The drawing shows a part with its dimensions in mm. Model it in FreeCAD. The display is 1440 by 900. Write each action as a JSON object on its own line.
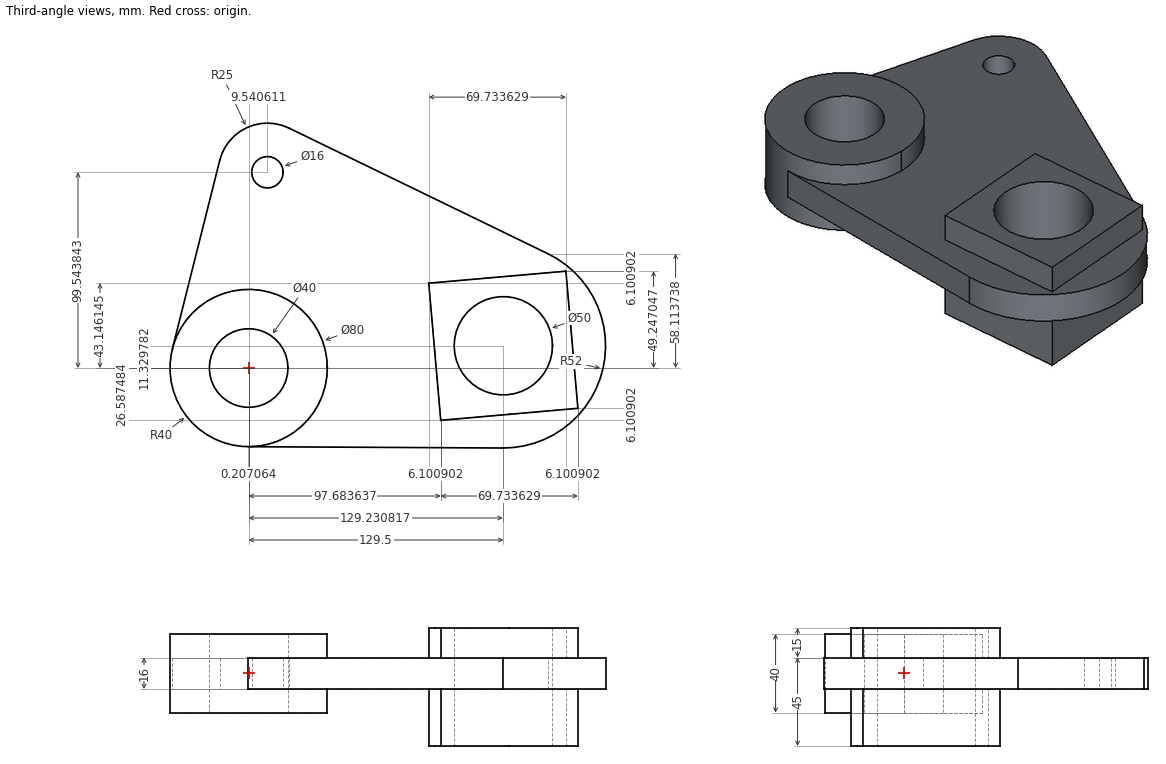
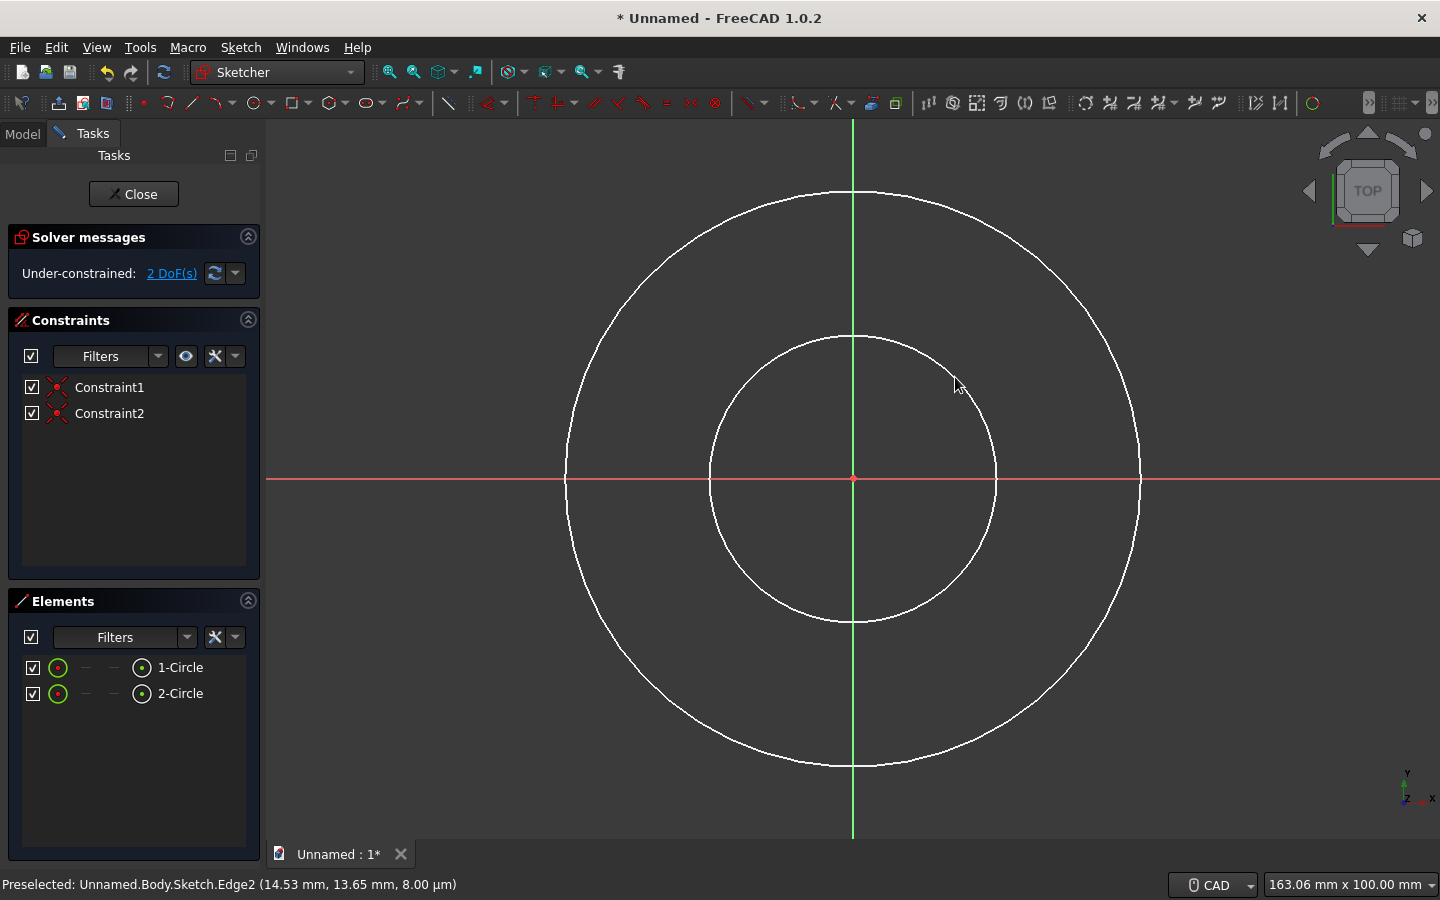
{"action": "key", "text": "d"}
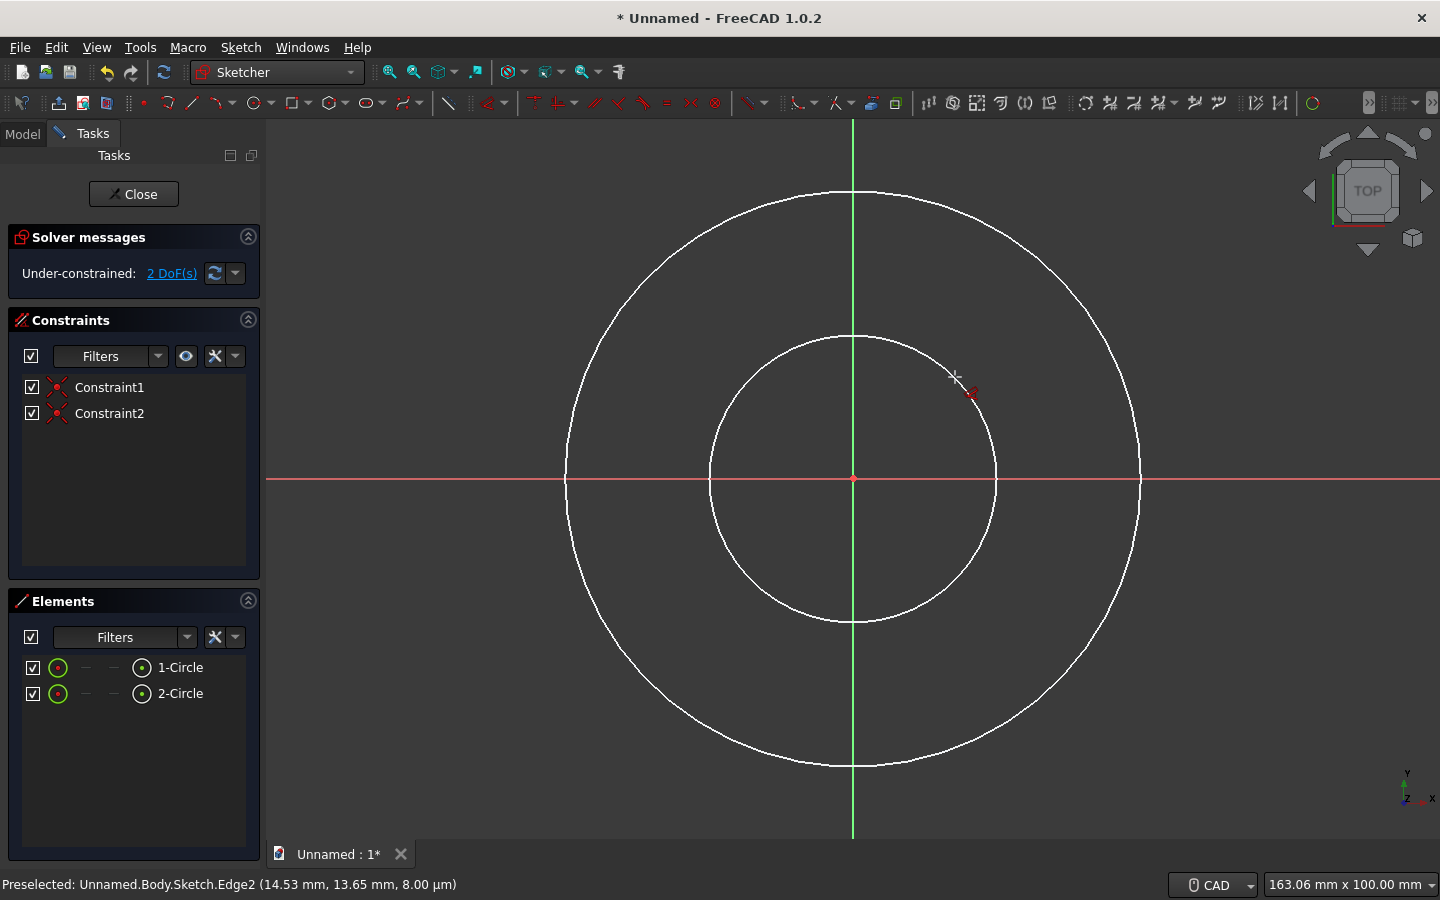
{"action": "left_click", "coordinate": [1056, 275]}
{"action": "left_click", "coordinate": [1079, 252]}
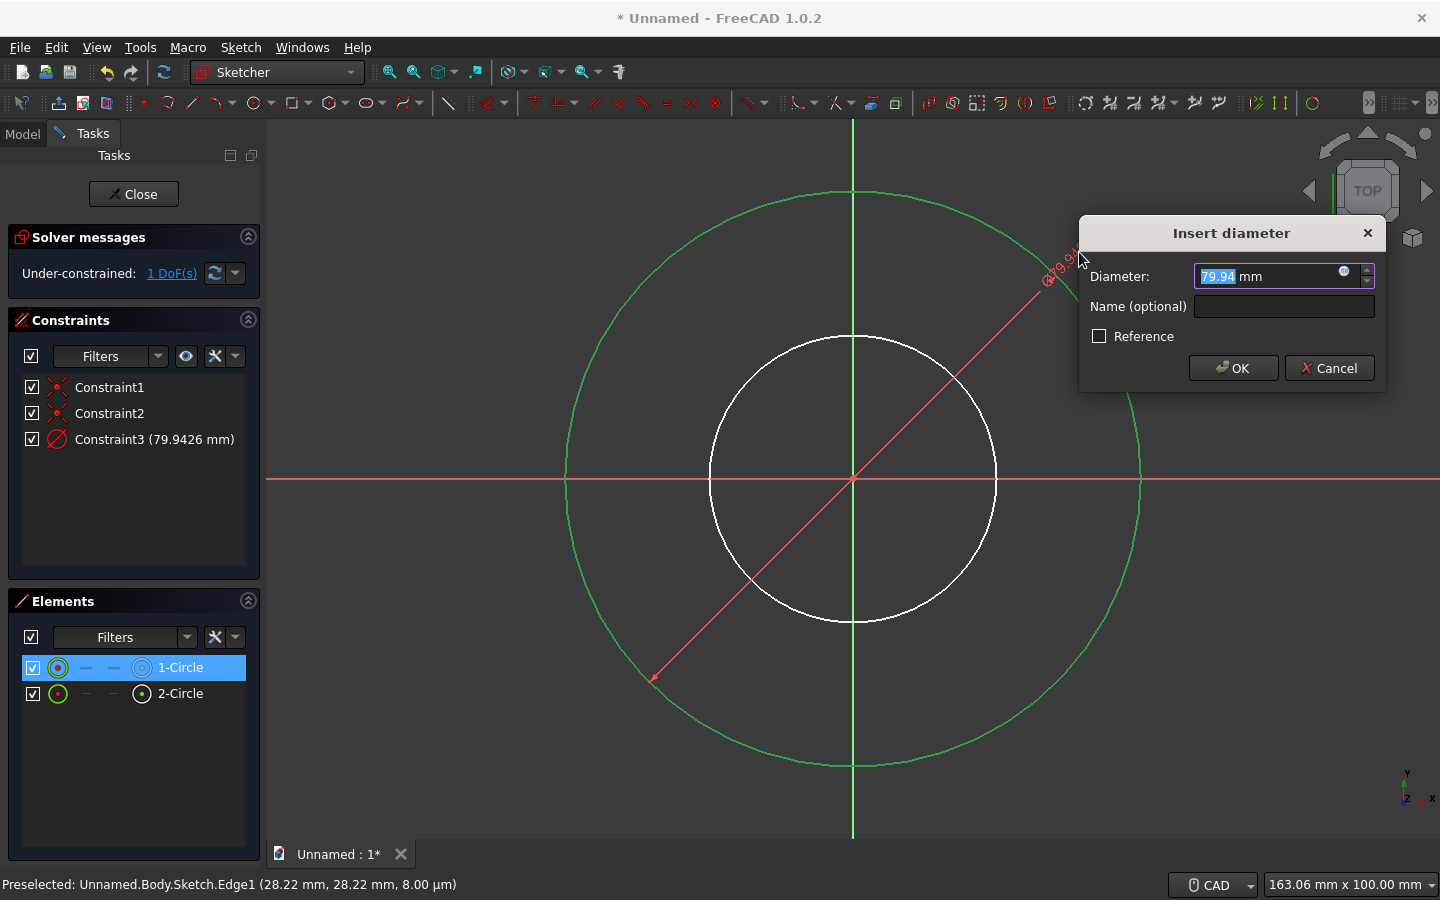
{"action": "type", "text": "80"}
{"action": "key", "text": "Return"}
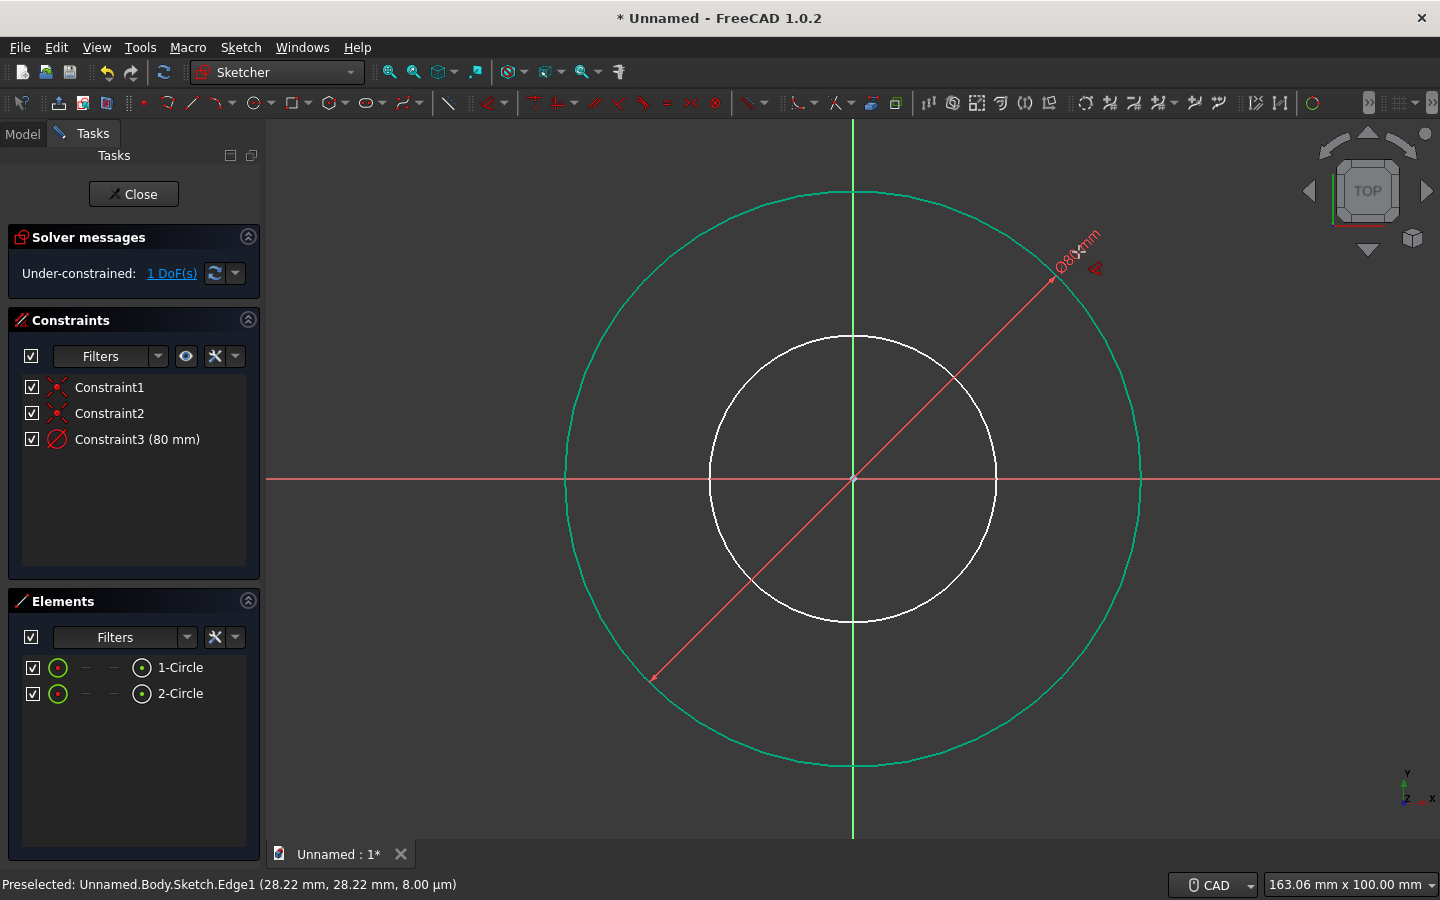
{"action": "left_click", "coordinate": [954, 377]}
{"action": "left_click", "coordinate": [977, 354]}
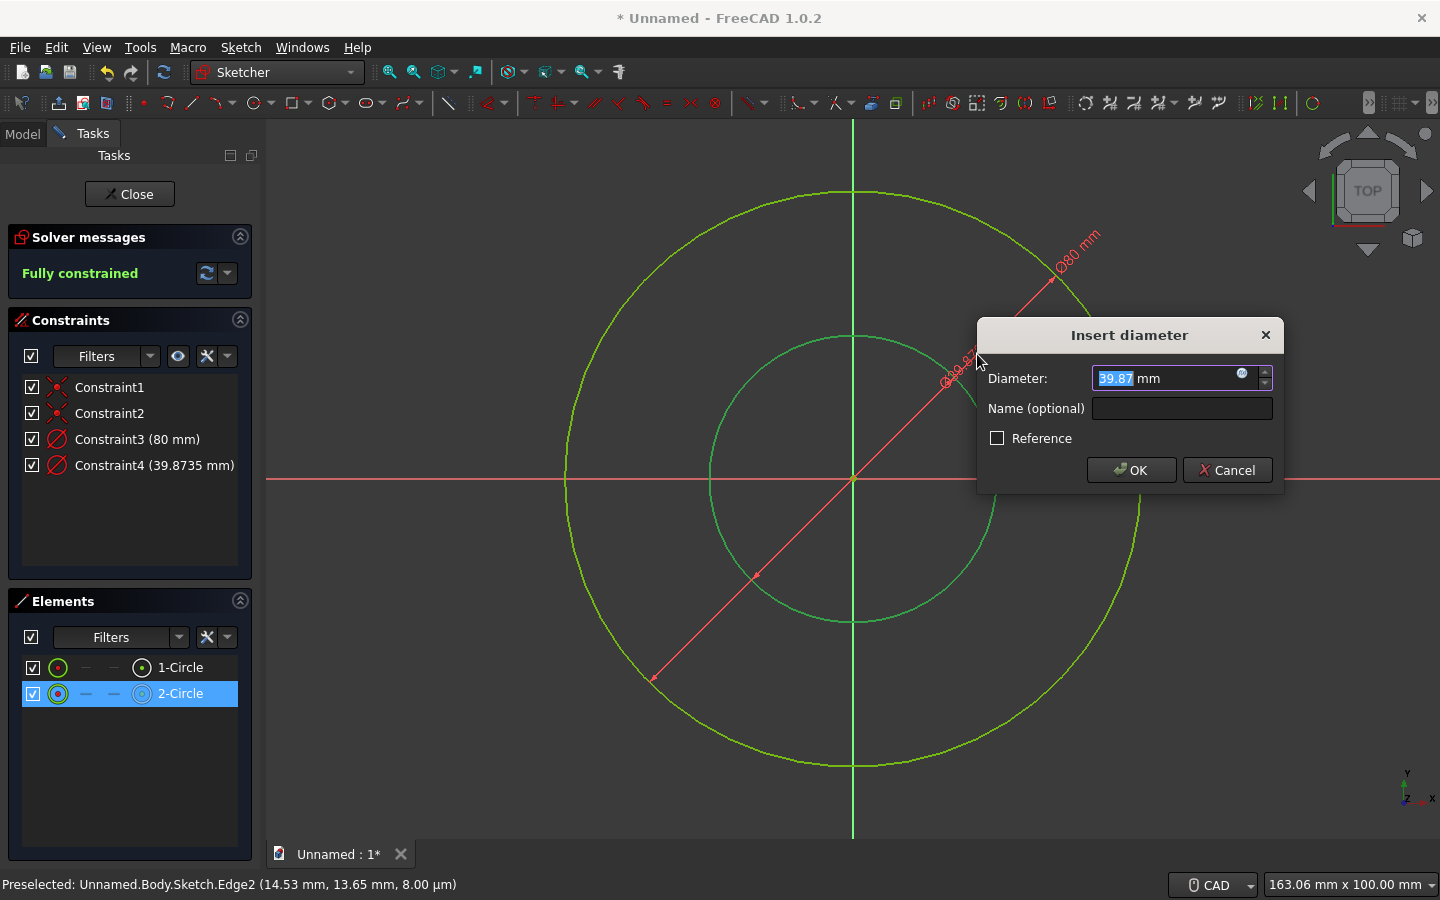
{"action": "type", "text": "40"}
{"action": "key", "text": "Return"}
{"action": "key", "text": "Escape"}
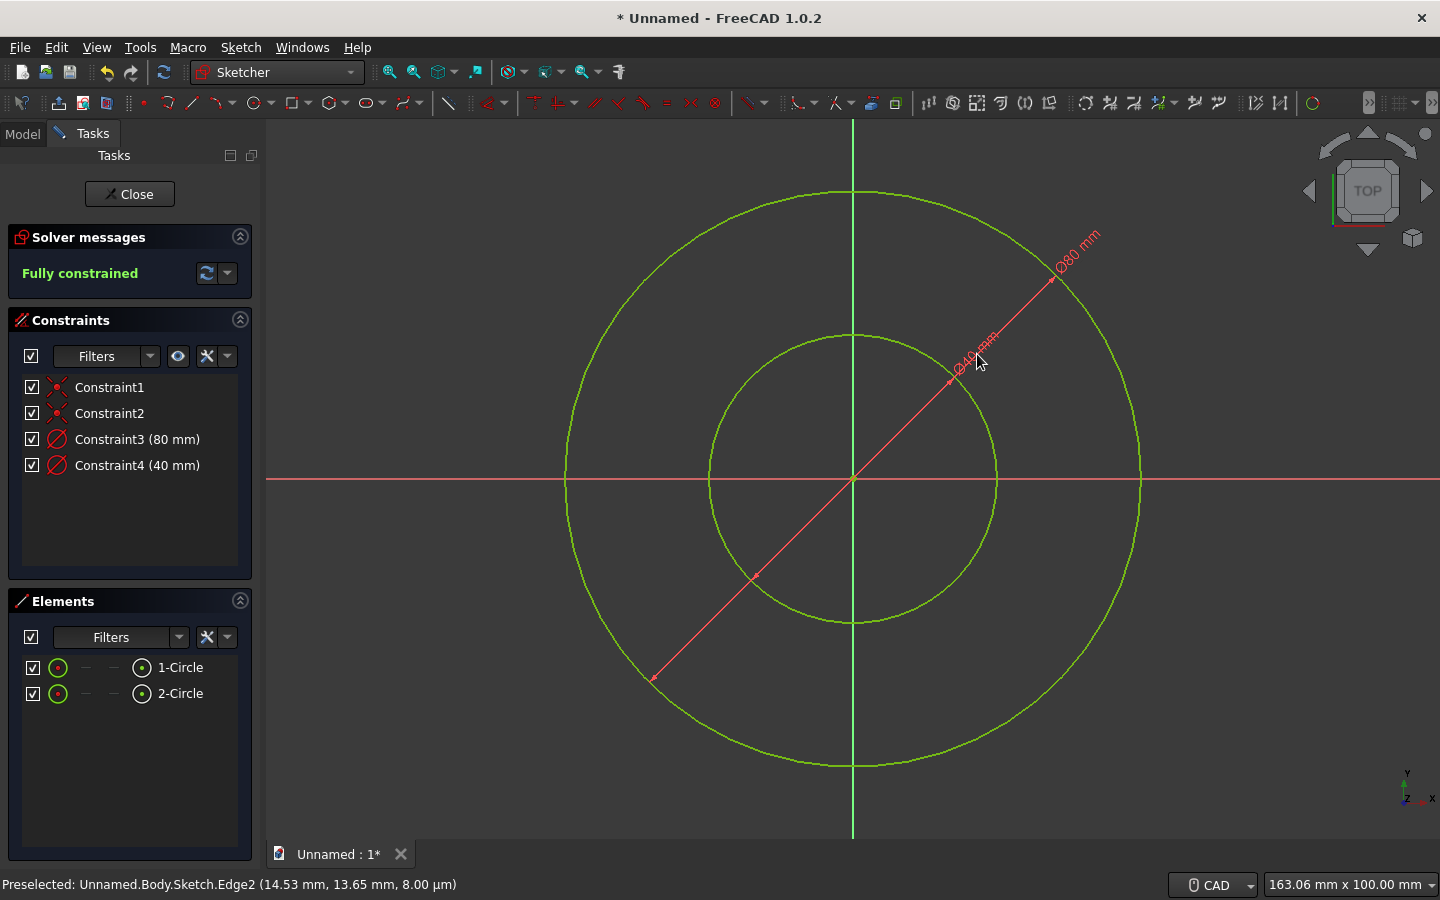
{"action": "left_click", "coordinate": [130, 194]}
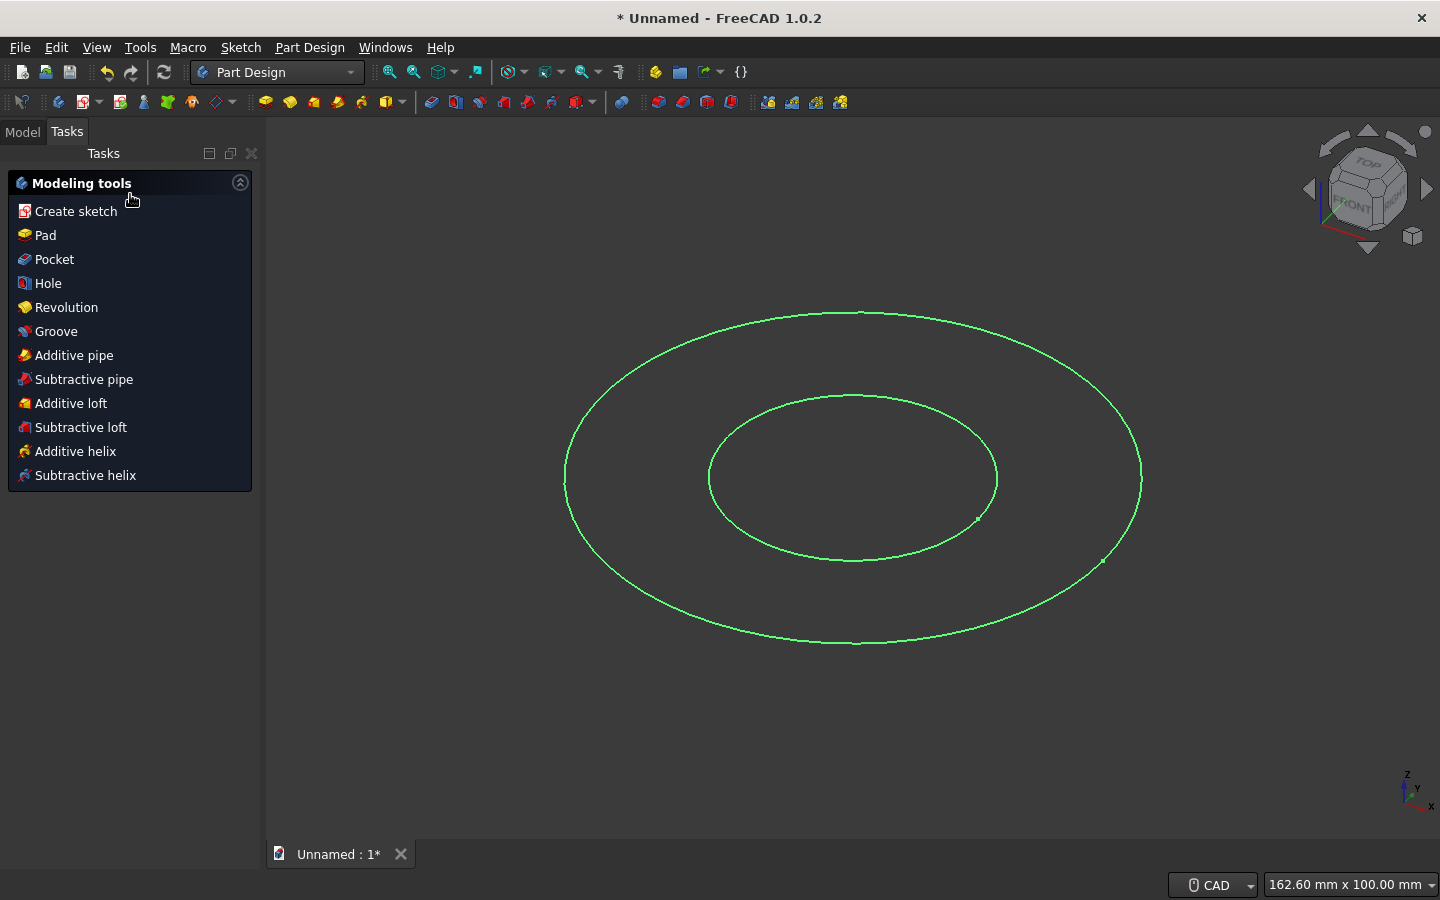
{"action": "left_click", "coordinate": [266, 102]}